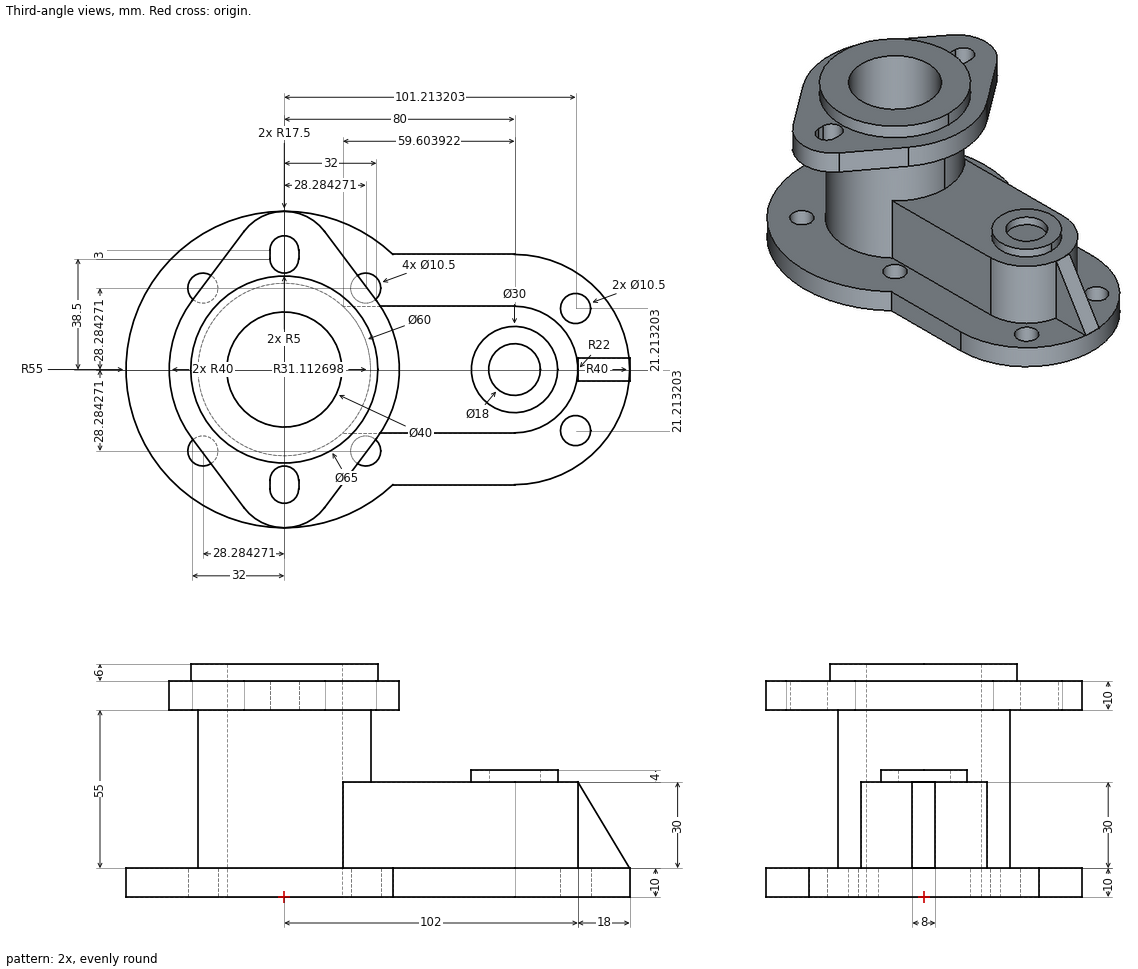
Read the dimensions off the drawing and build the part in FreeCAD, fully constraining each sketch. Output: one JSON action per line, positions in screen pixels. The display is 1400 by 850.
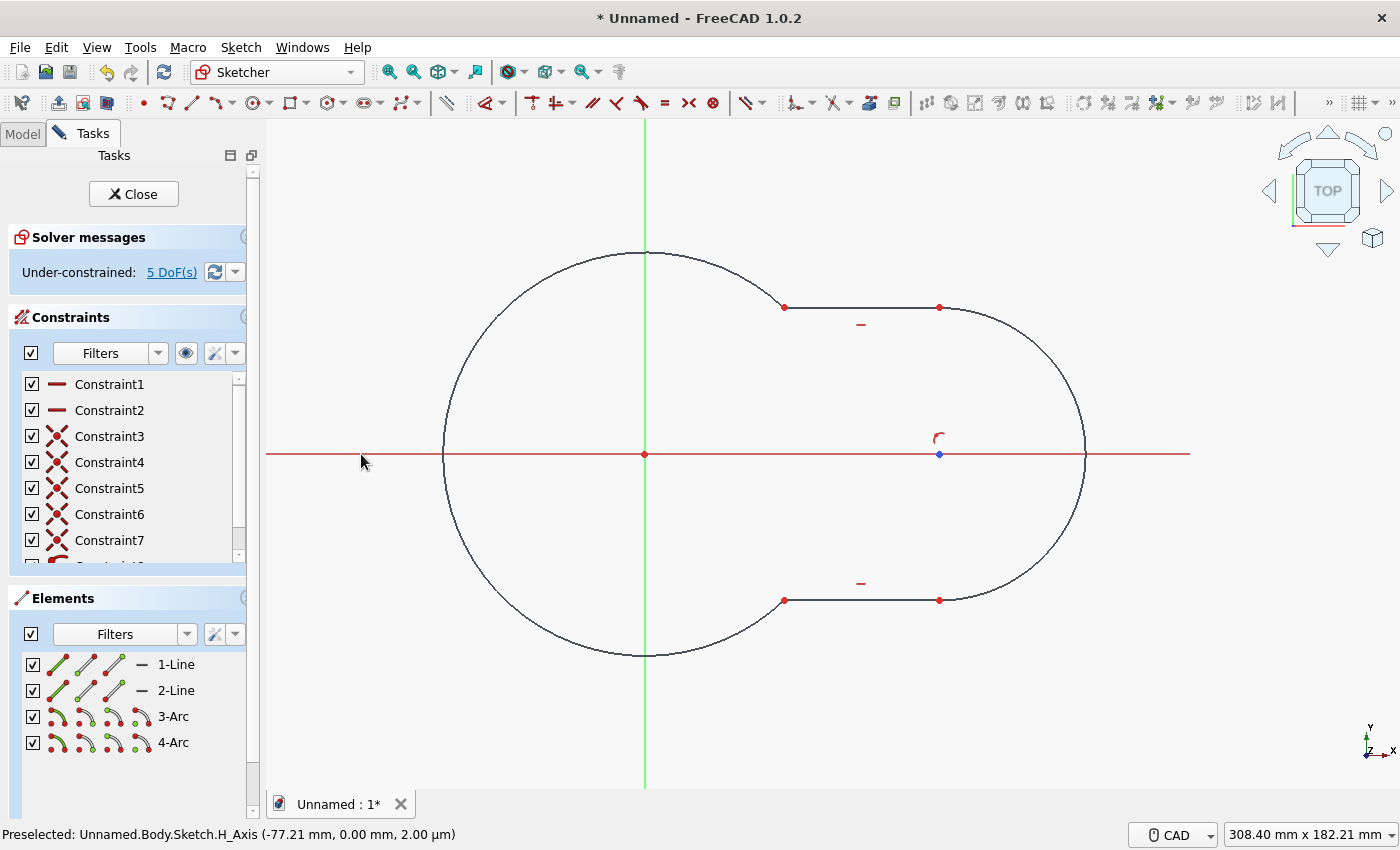
{"action": "key", "text": "d"}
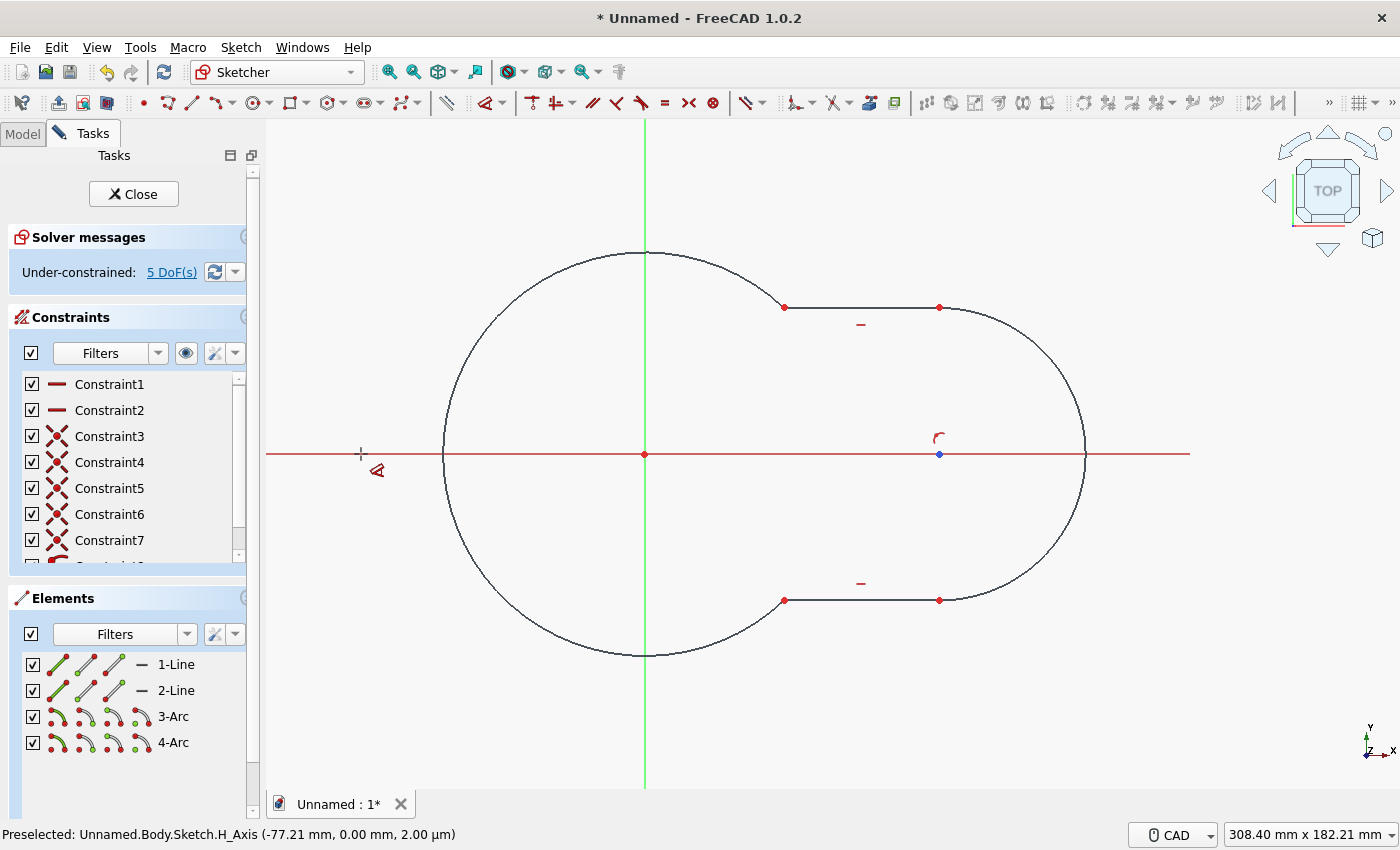
{"action": "left_click", "coordinate": [525, 292]}
{"action": "left_click", "coordinate": [506, 266]}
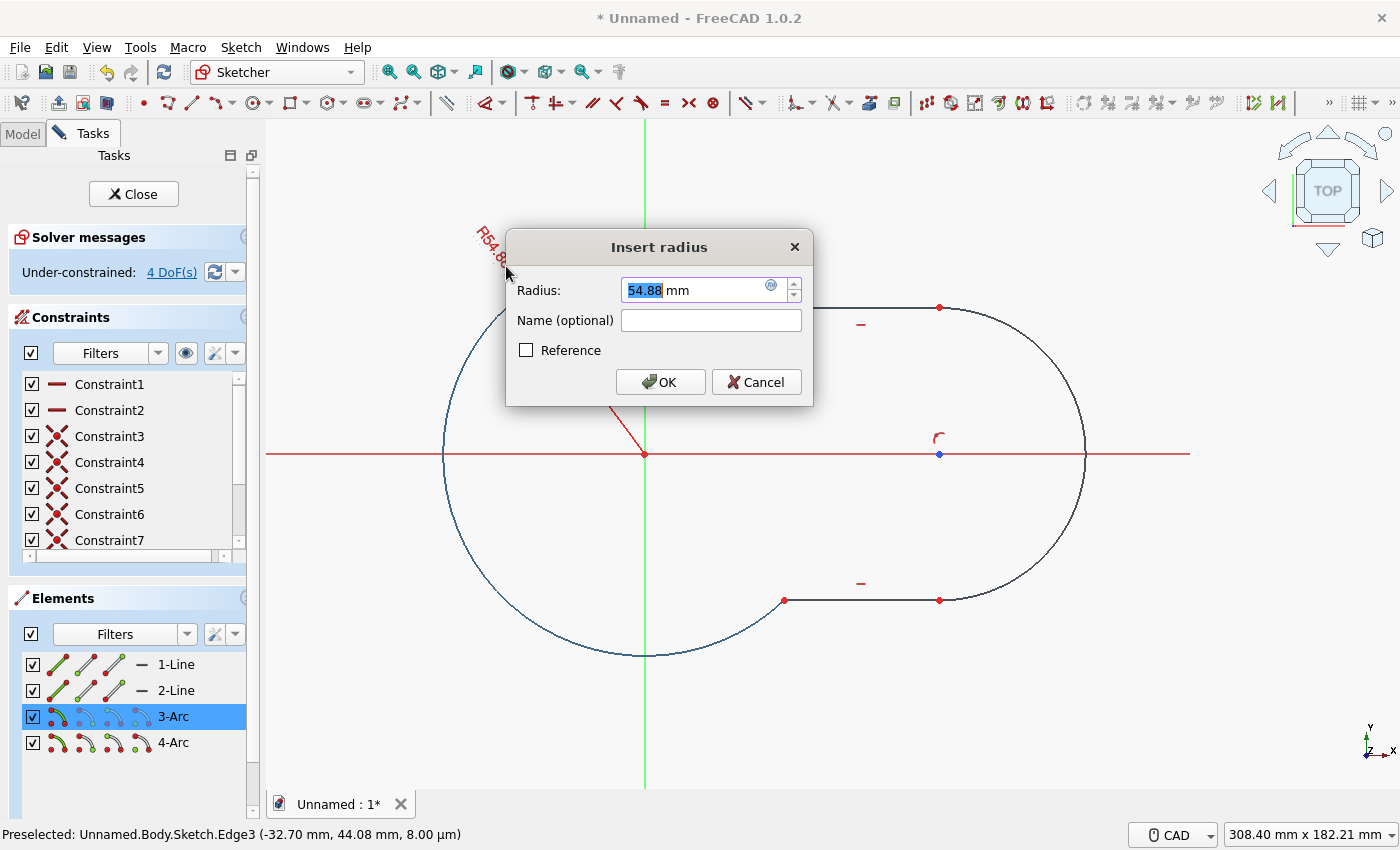
{"action": "type", "text": "55"}
{"action": "key", "text": "Return"}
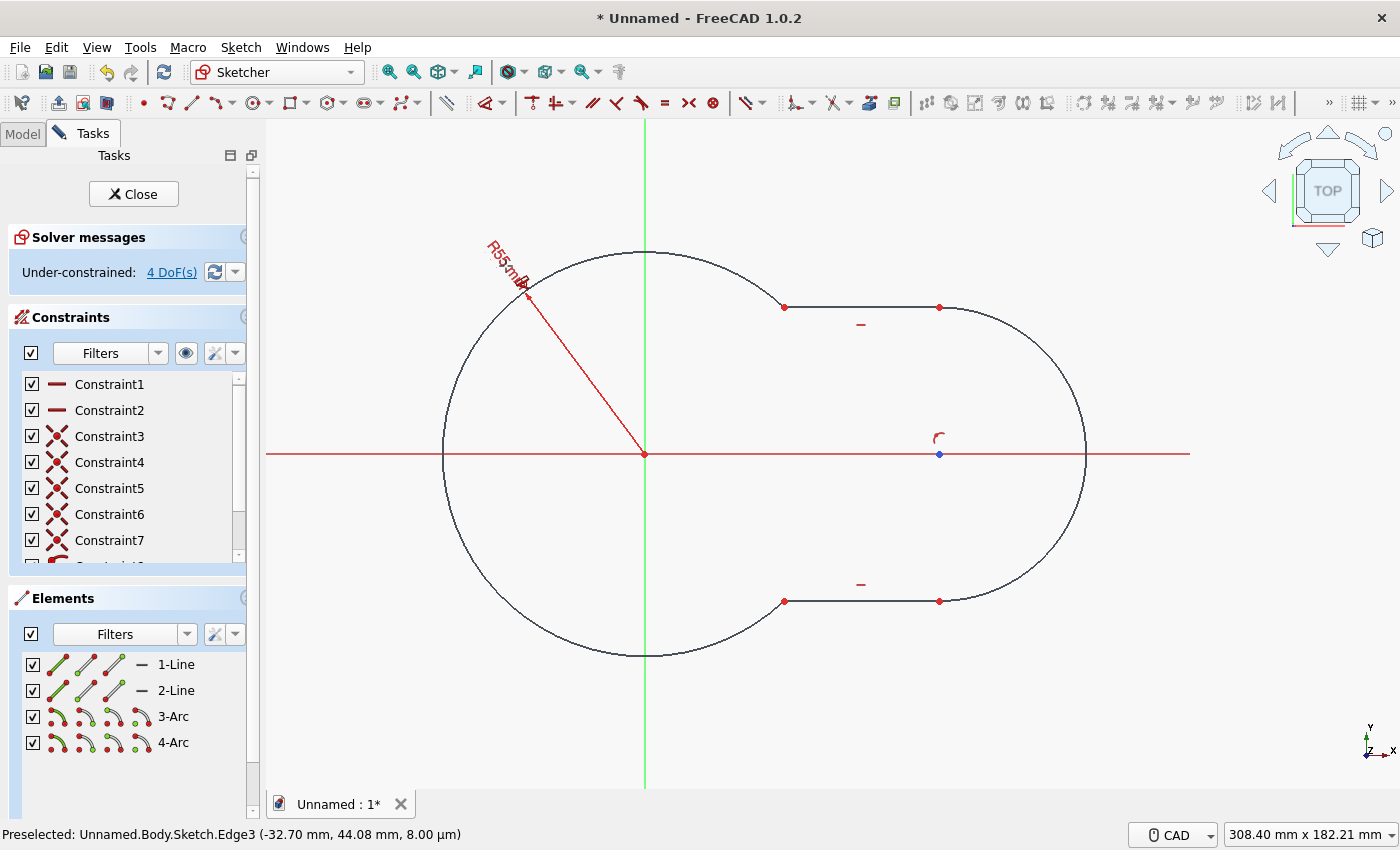
{"action": "left_click", "coordinate": [1058, 541]}
{"action": "left_click", "coordinate": [1084, 560]}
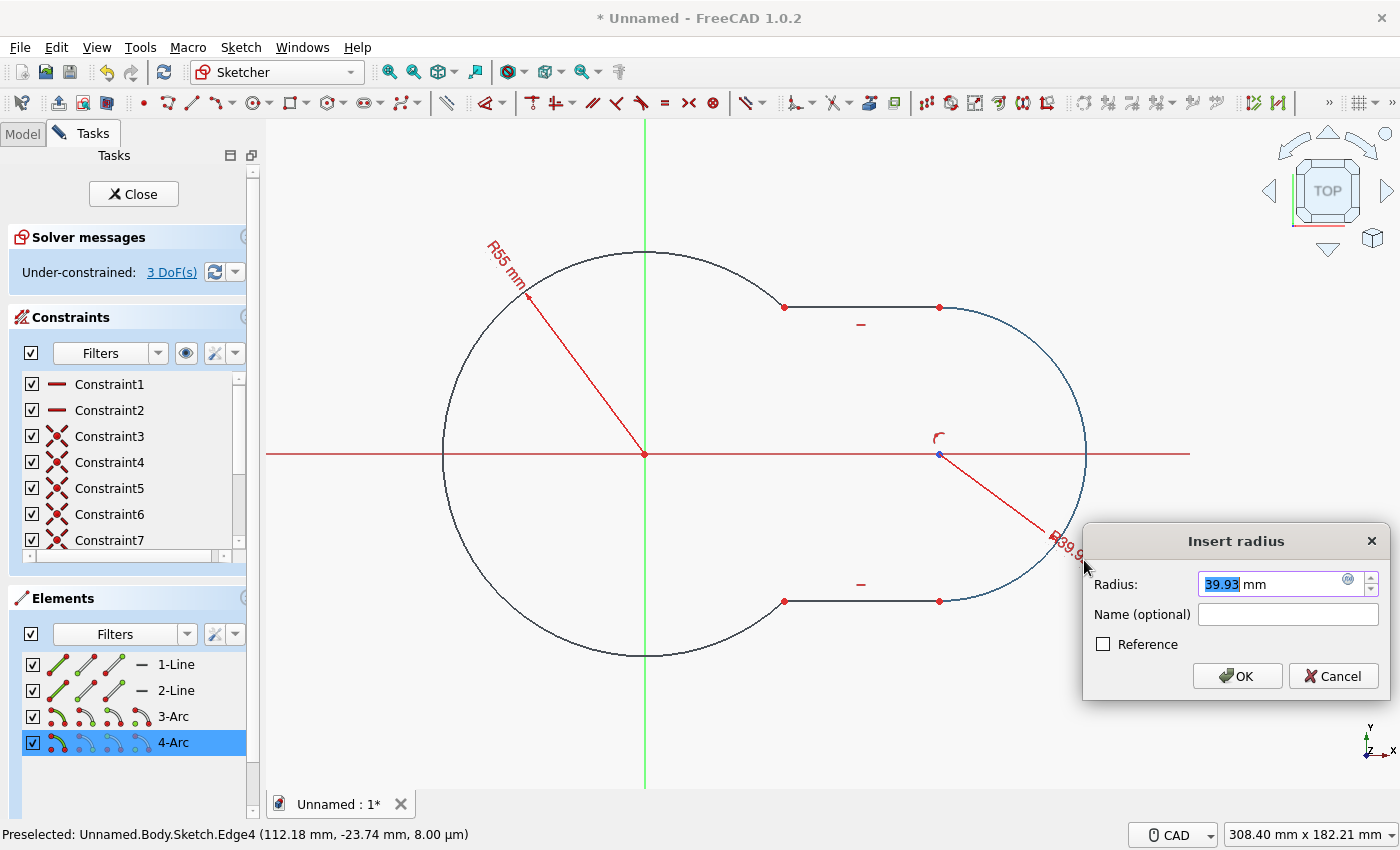
{"action": "type", "text": "40"}
{"action": "key", "text": "Return"}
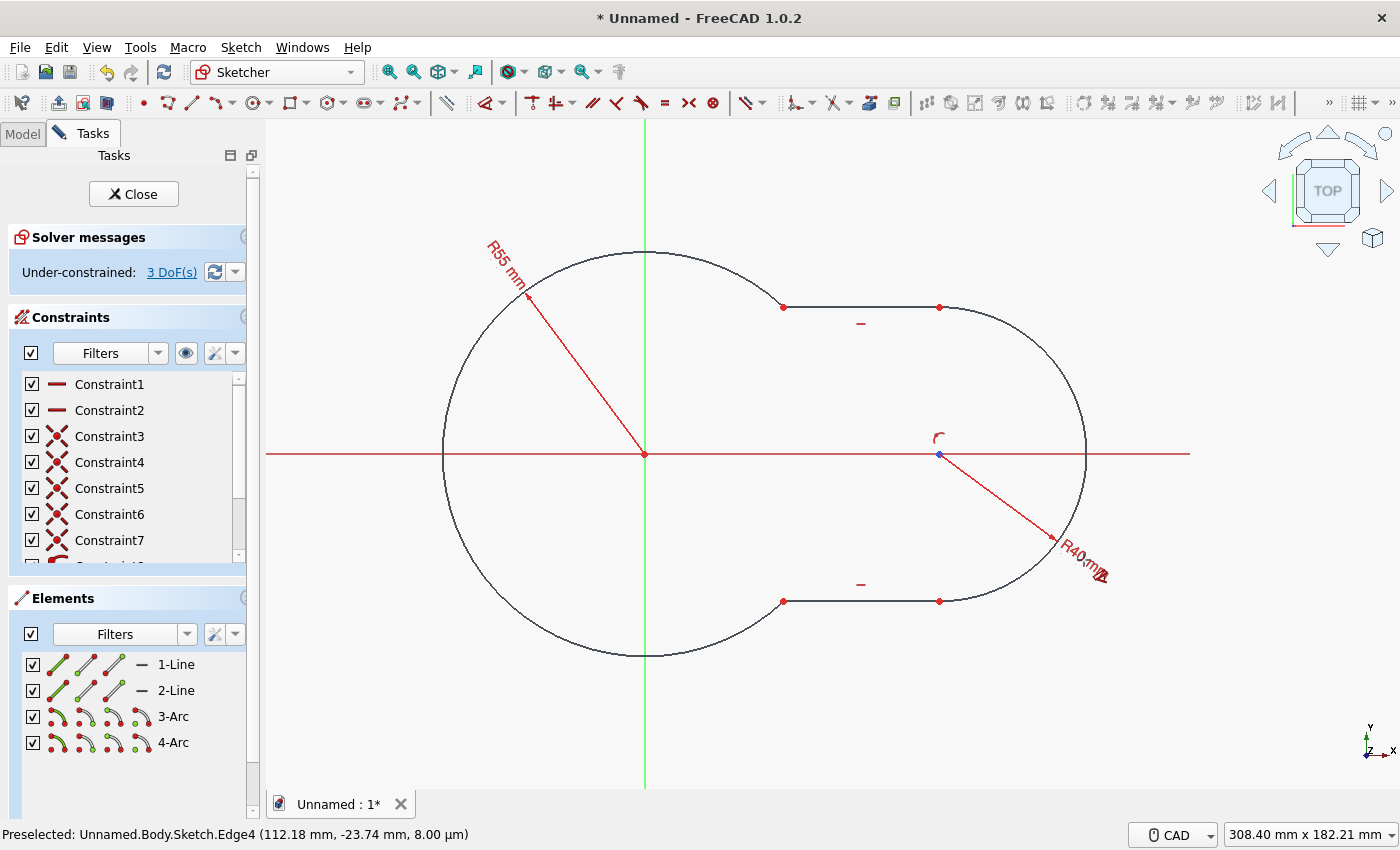
{"action": "left_click", "coordinate": [939, 307]}
{"action": "left_click", "coordinate": [792, 273]}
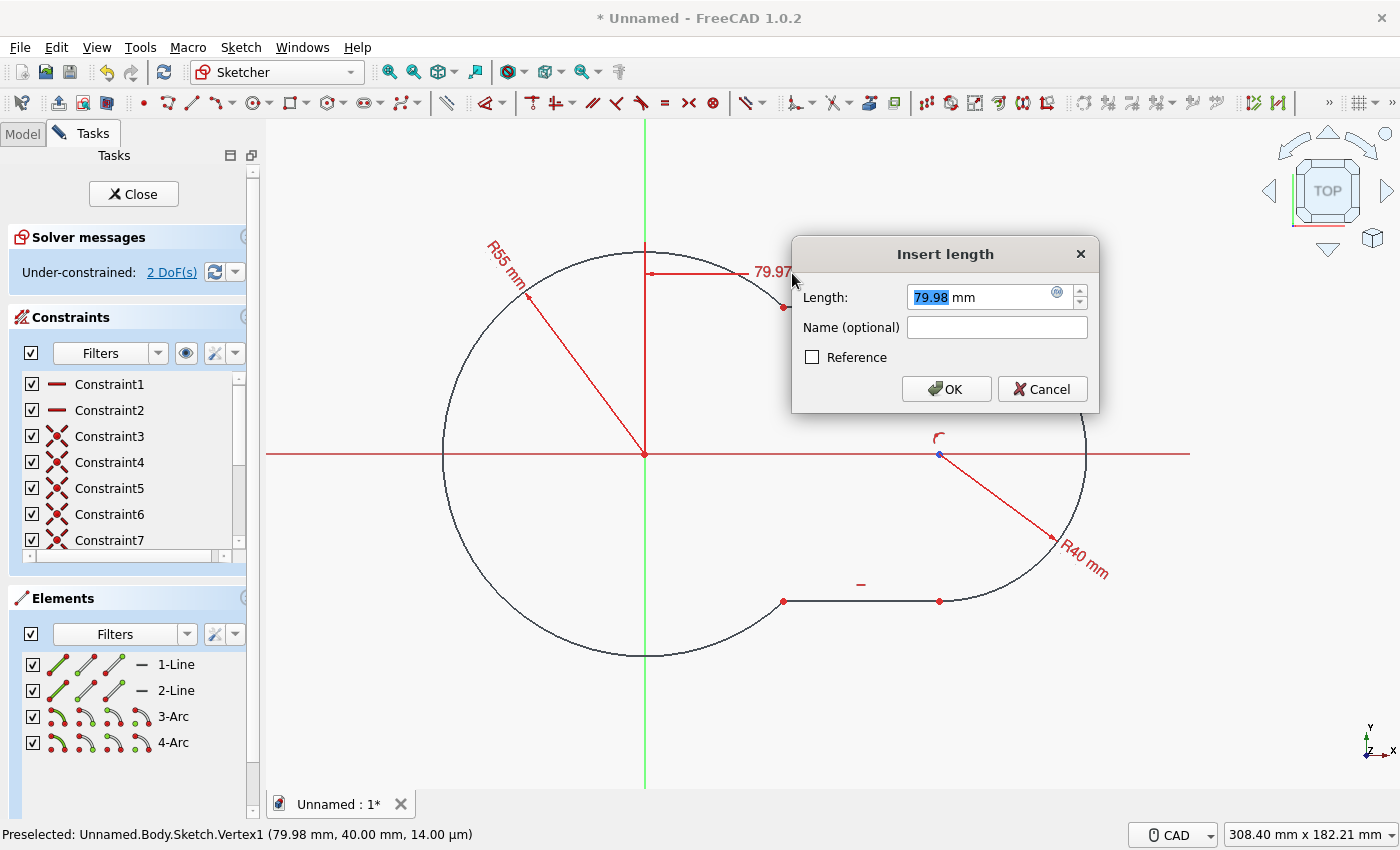
{"action": "type", "text": "80"}
{"action": "key", "text": "Return"}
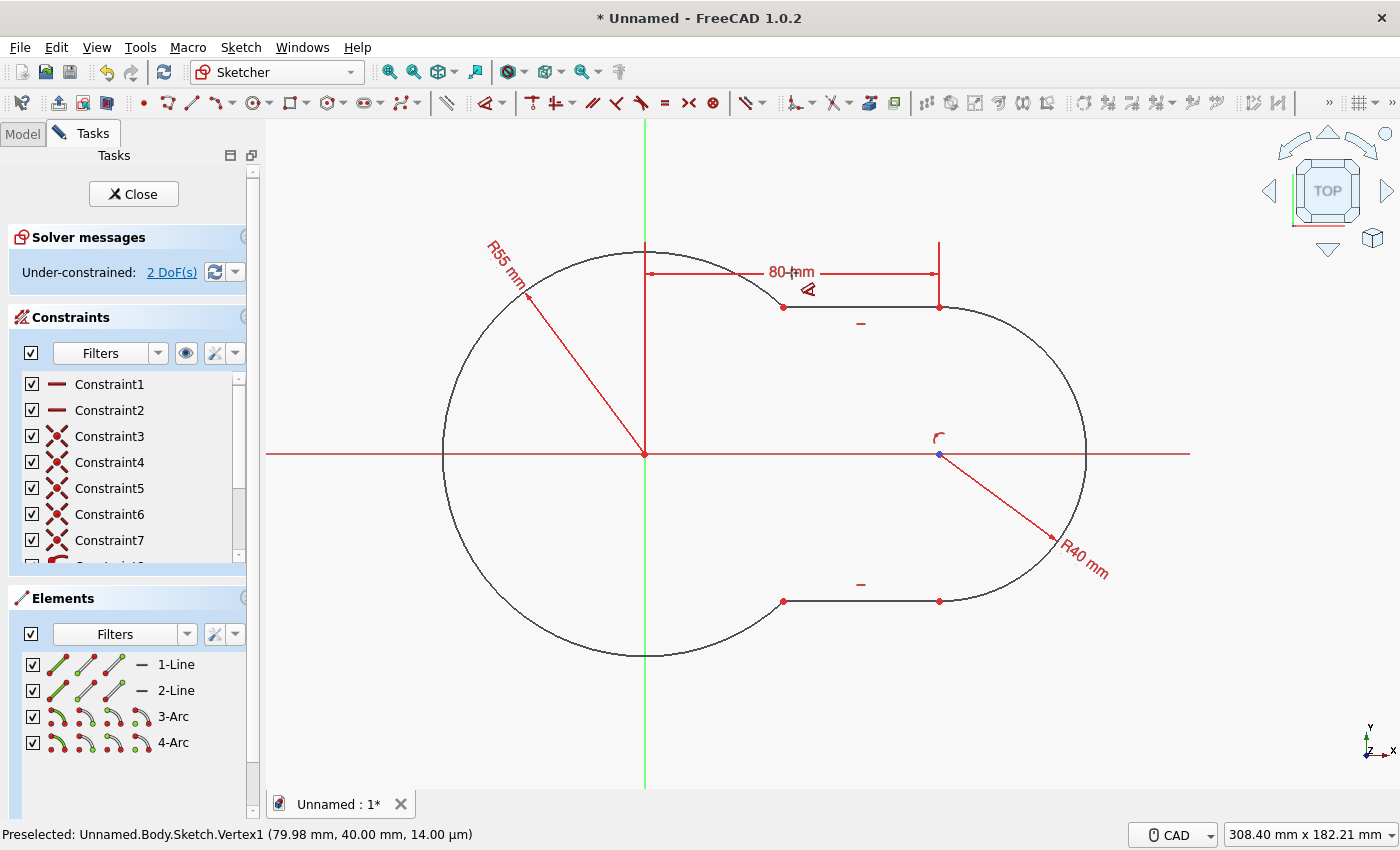
{"action": "left_click", "coordinate": [939, 601]}
{"action": "left_click", "coordinate": [792, 635]}